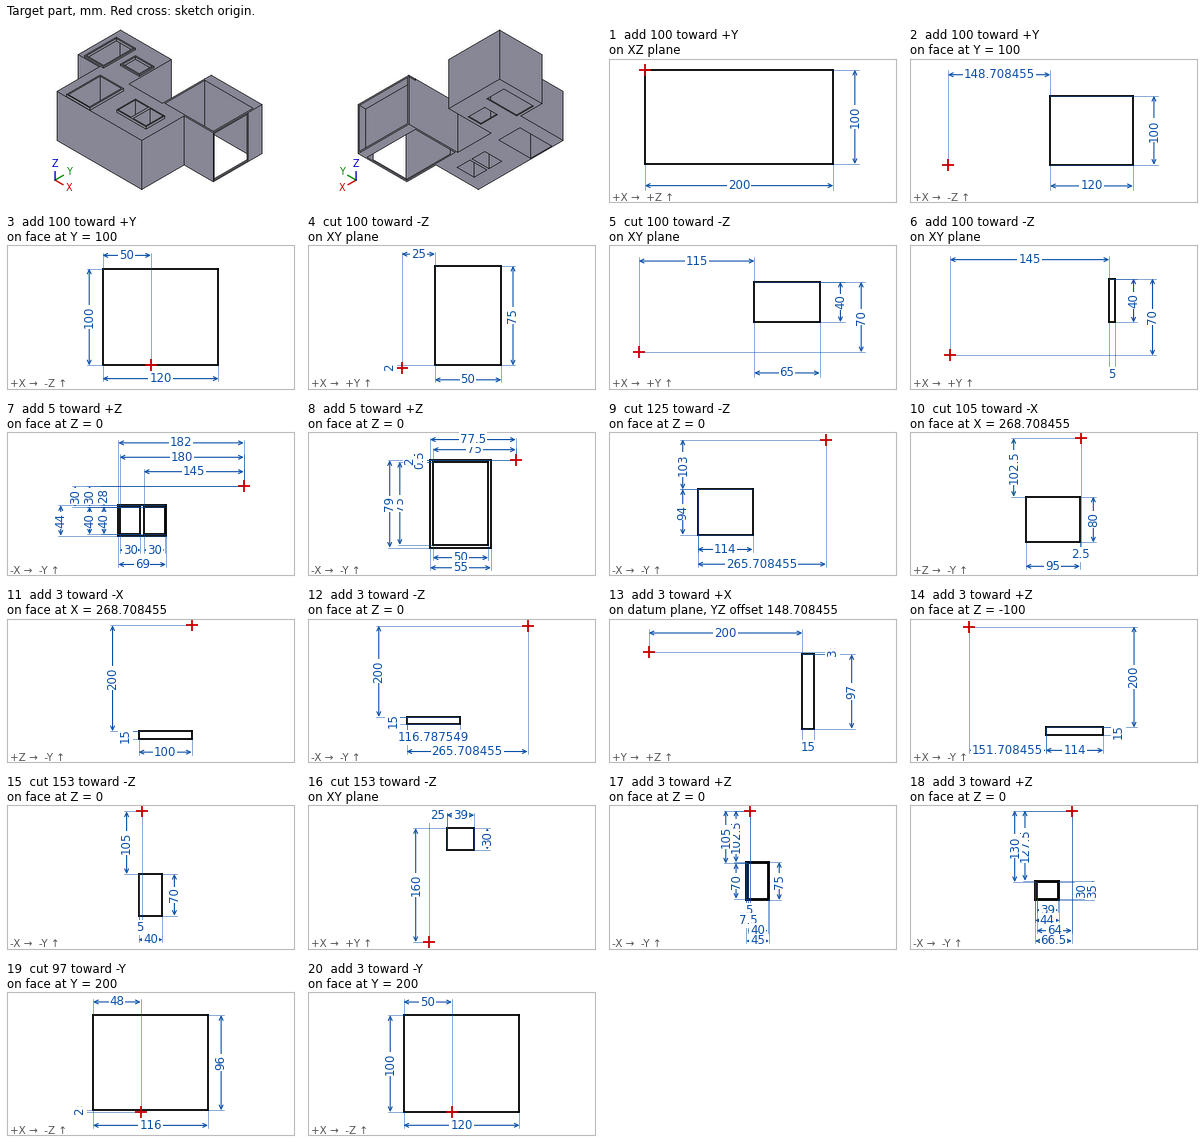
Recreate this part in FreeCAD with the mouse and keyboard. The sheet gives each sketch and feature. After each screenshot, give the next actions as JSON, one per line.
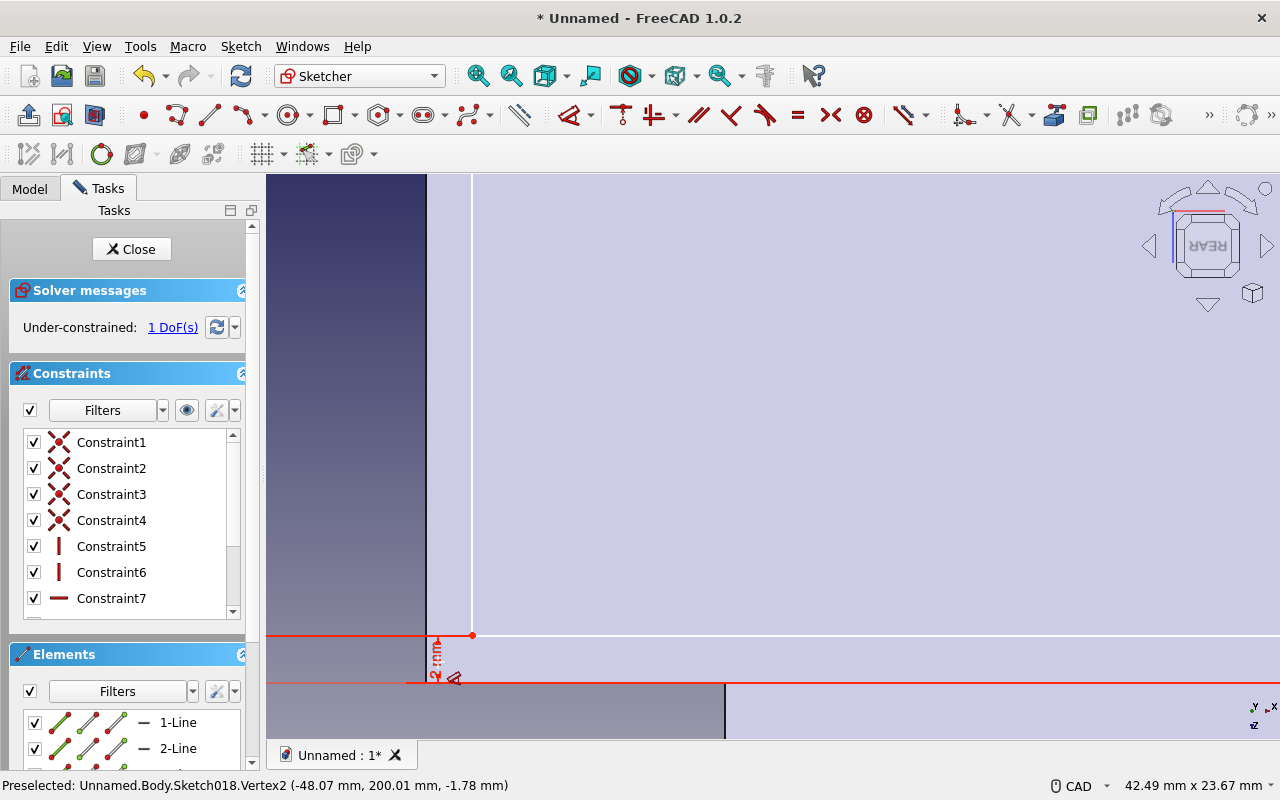
{"action": "scroll", "coordinate": [476, 643], "scroll_direction": "down", "scroll_amount": 9}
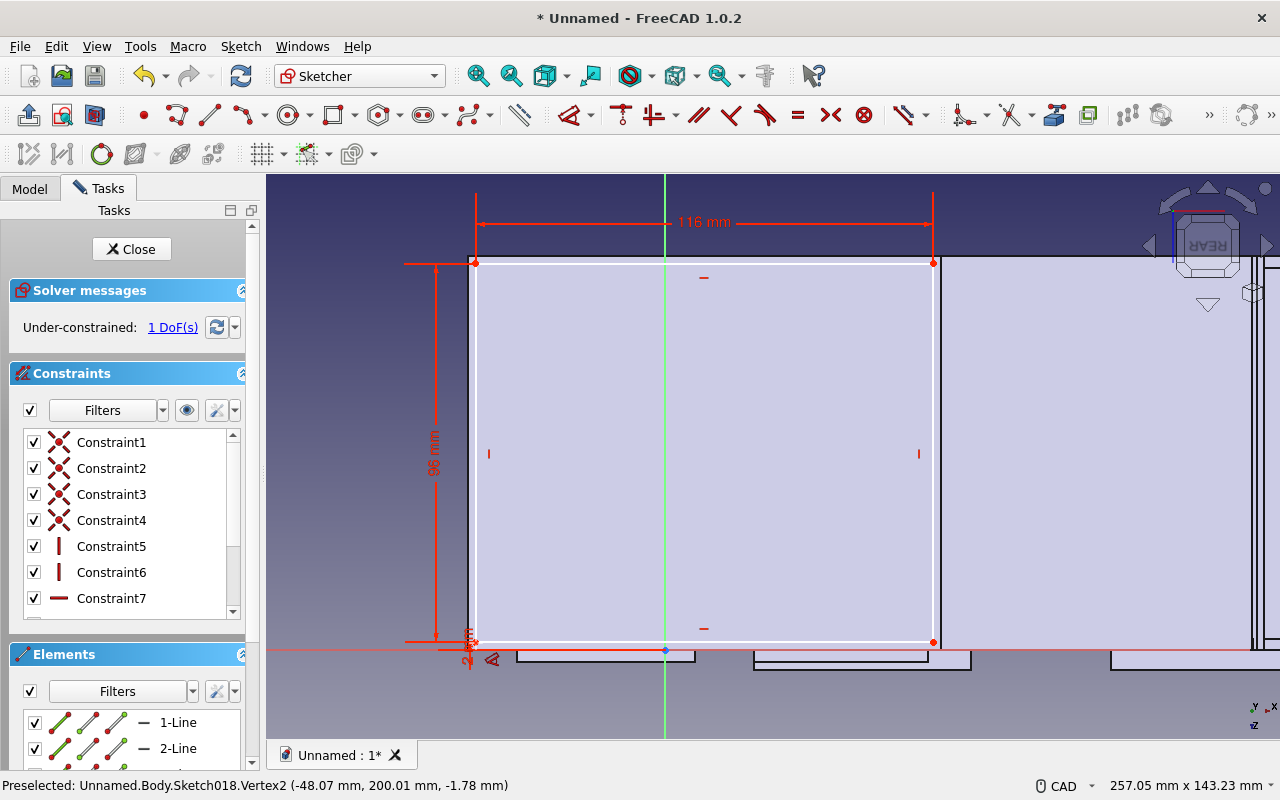
{"action": "left_click", "coordinate": [476, 264]}
{"action": "left_click", "coordinate": [570, 684]}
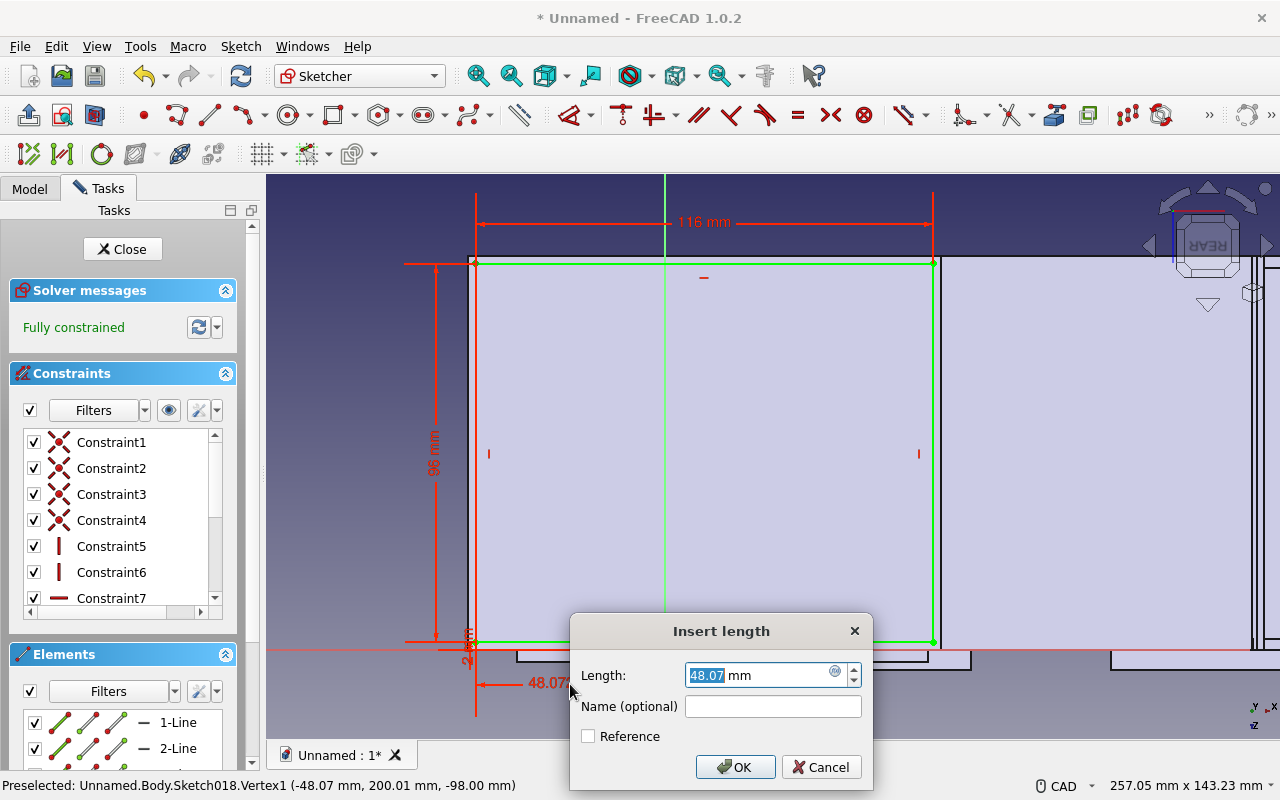
{"action": "type", "text": "48"}
{"action": "key", "text": "Return"}
{"action": "key", "text": "Escape"}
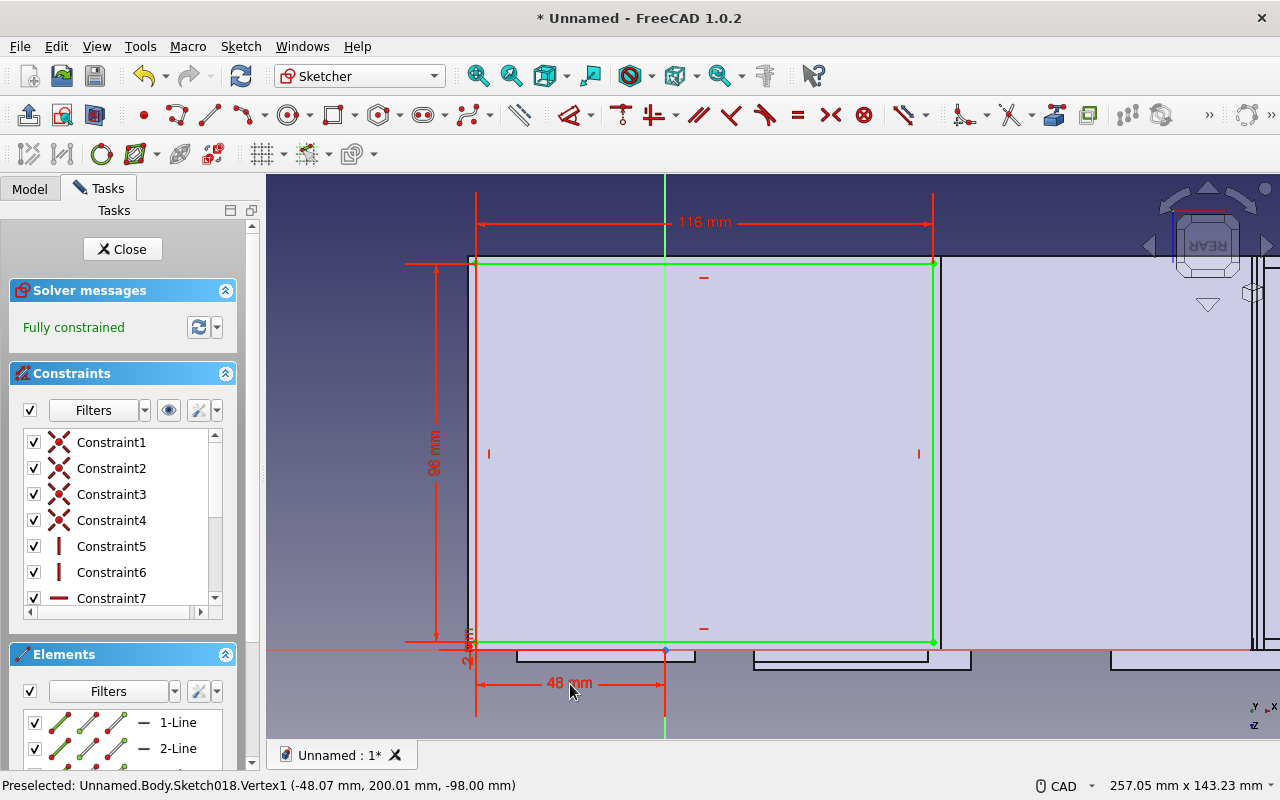
{"action": "left_click", "coordinate": [123, 249]}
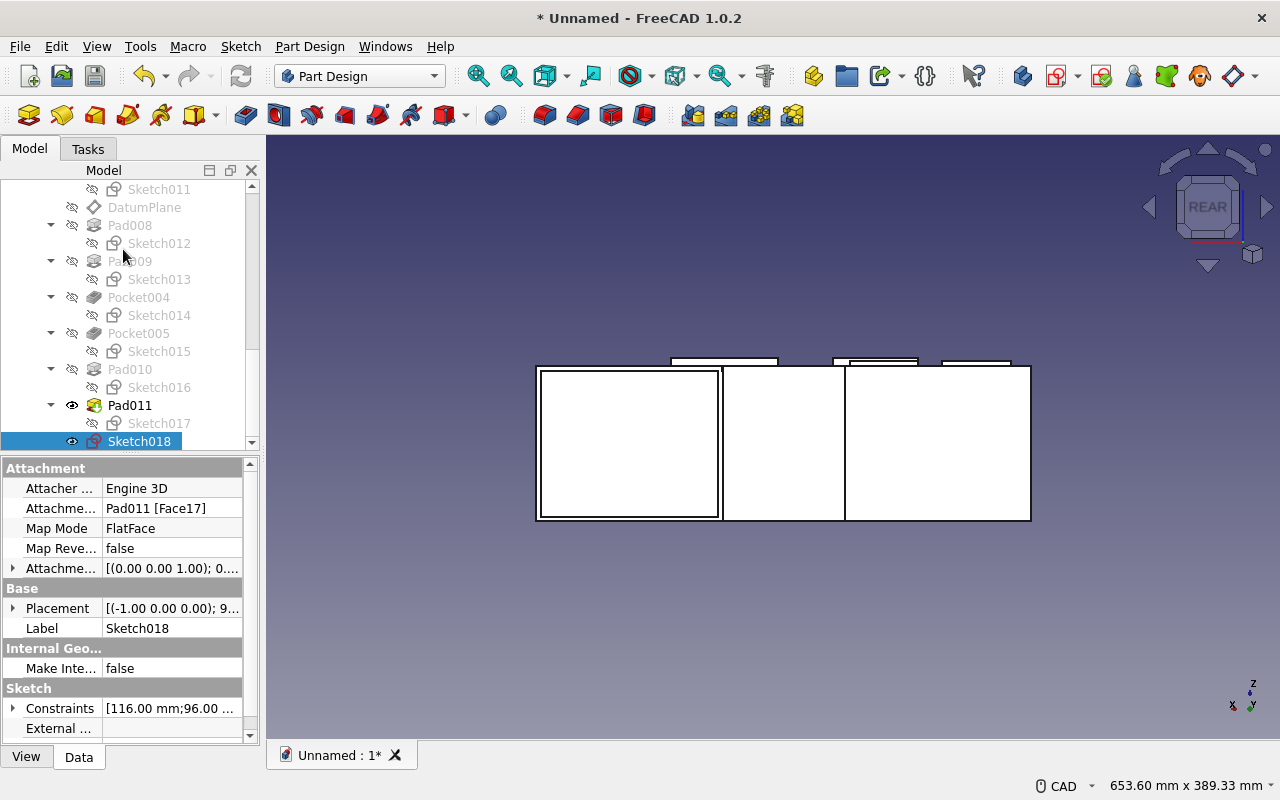
{"action": "left_click", "coordinate": [246, 116]}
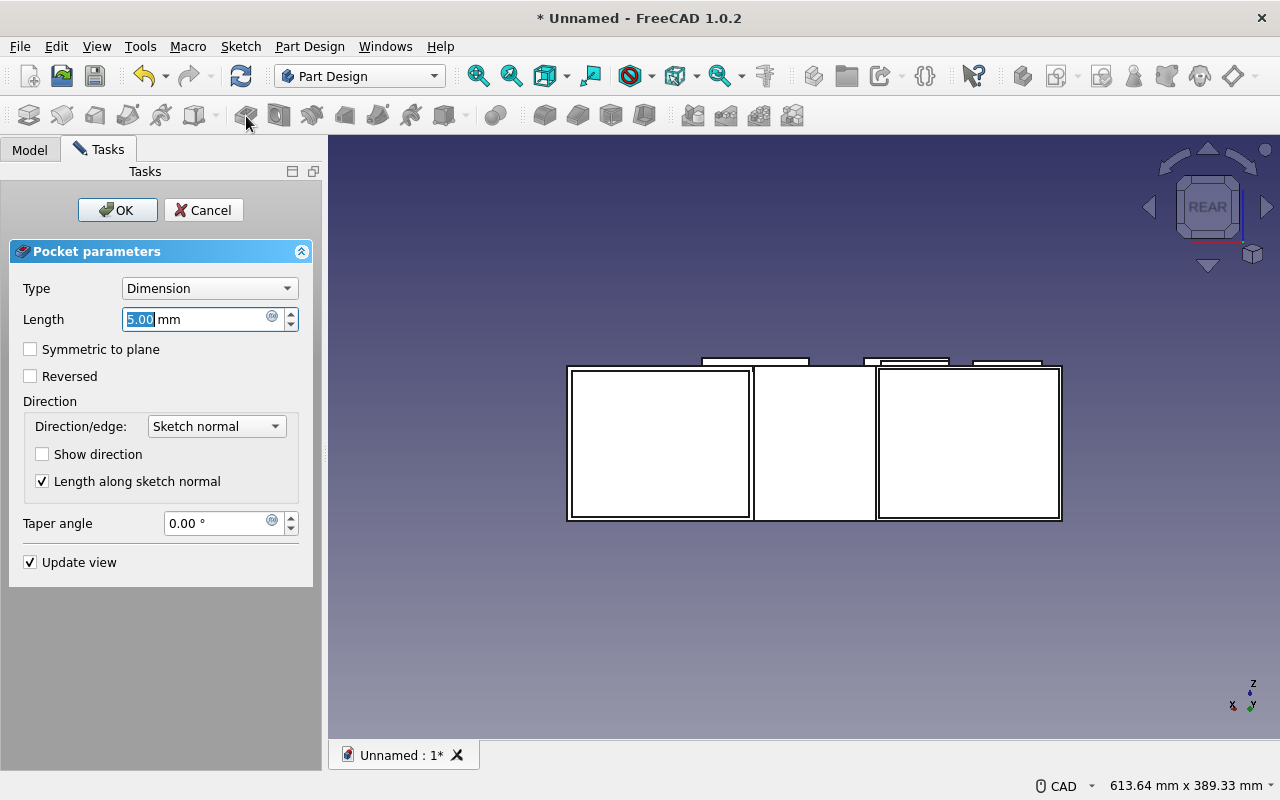
{"action": "type", "text": "97"}
{"action": "key", "text": "Tab"}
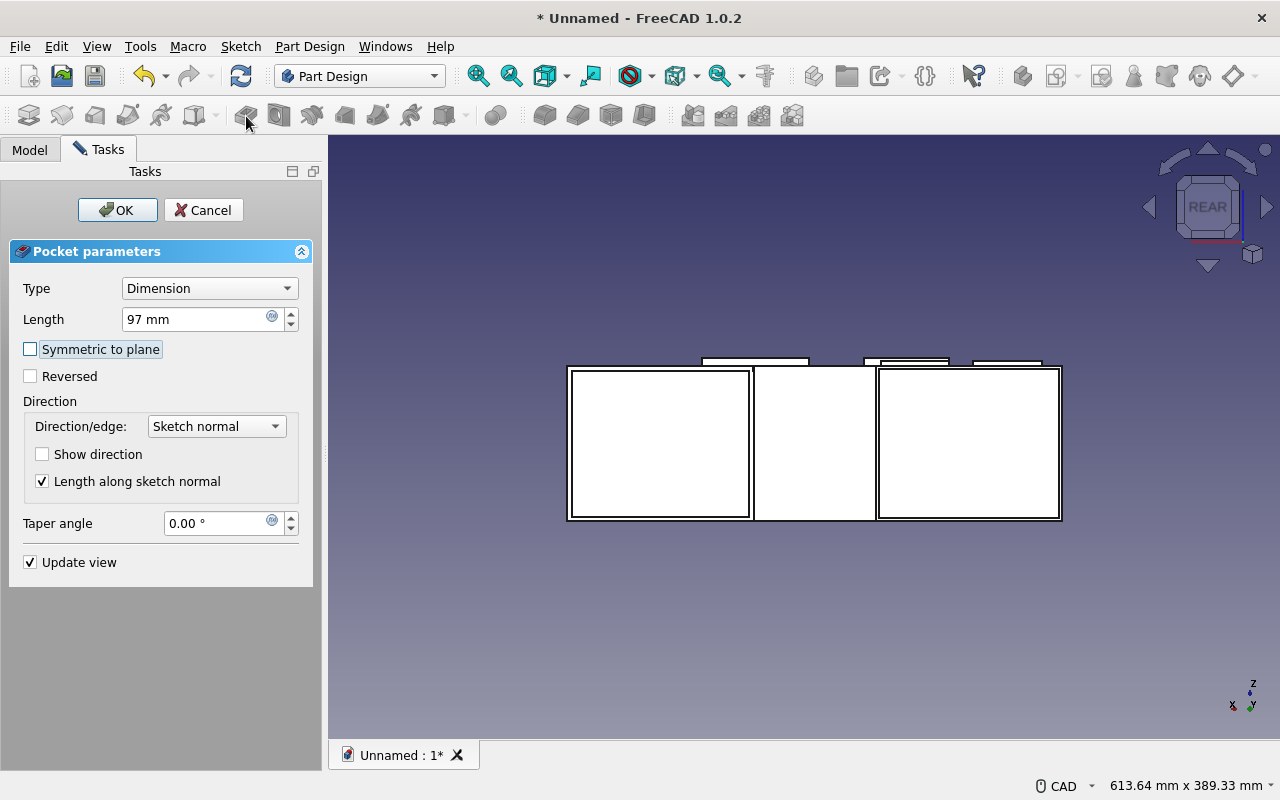
{"action": "left_click", "coordinate": [118, 210]}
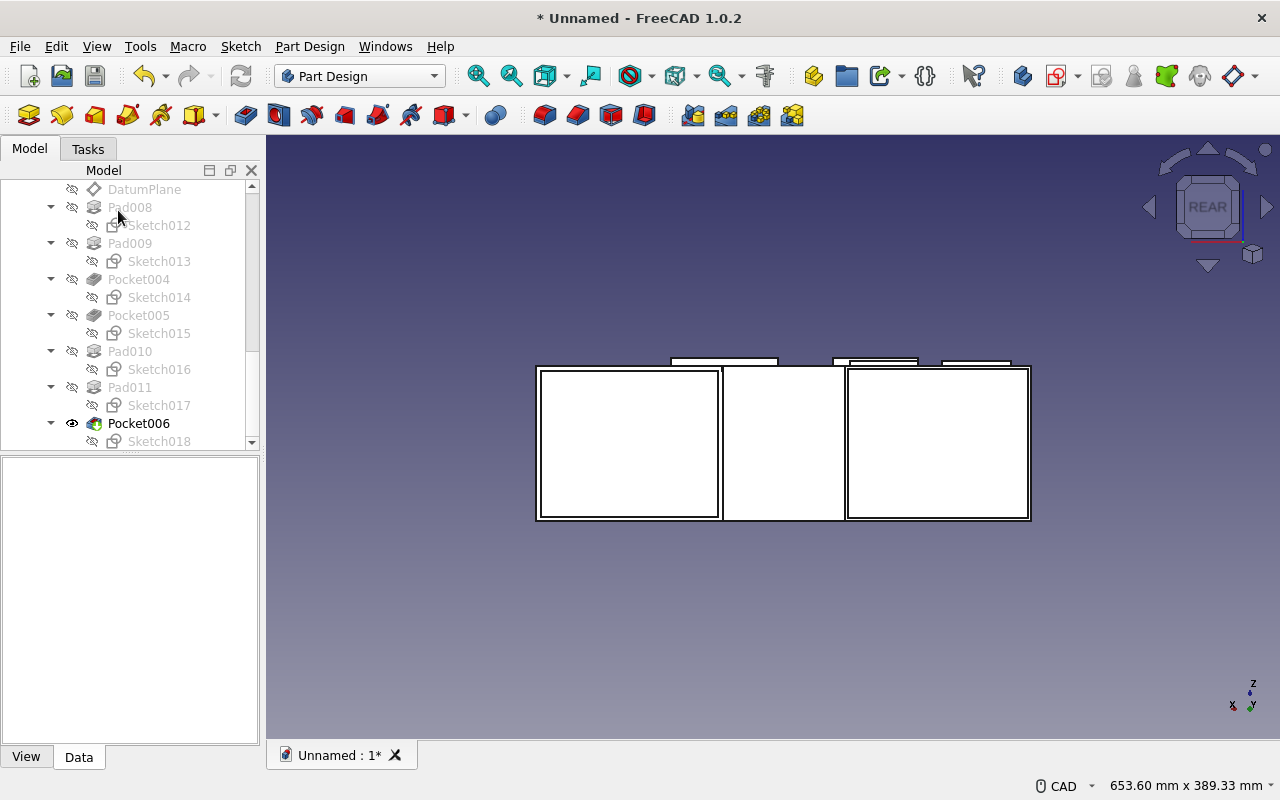
{"action": "left_click", "coordinate": [629, 443]}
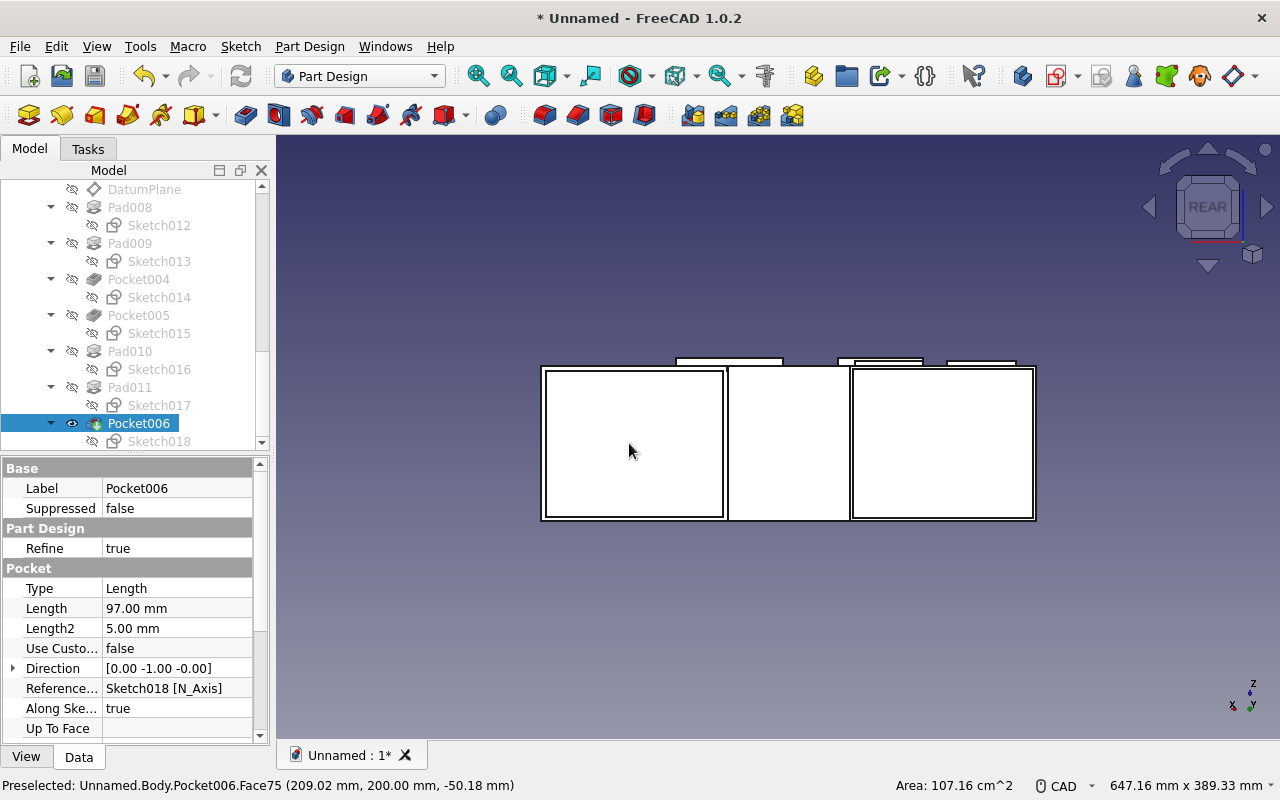
{"action": "left_click", "coordinate": [1056, 76]}